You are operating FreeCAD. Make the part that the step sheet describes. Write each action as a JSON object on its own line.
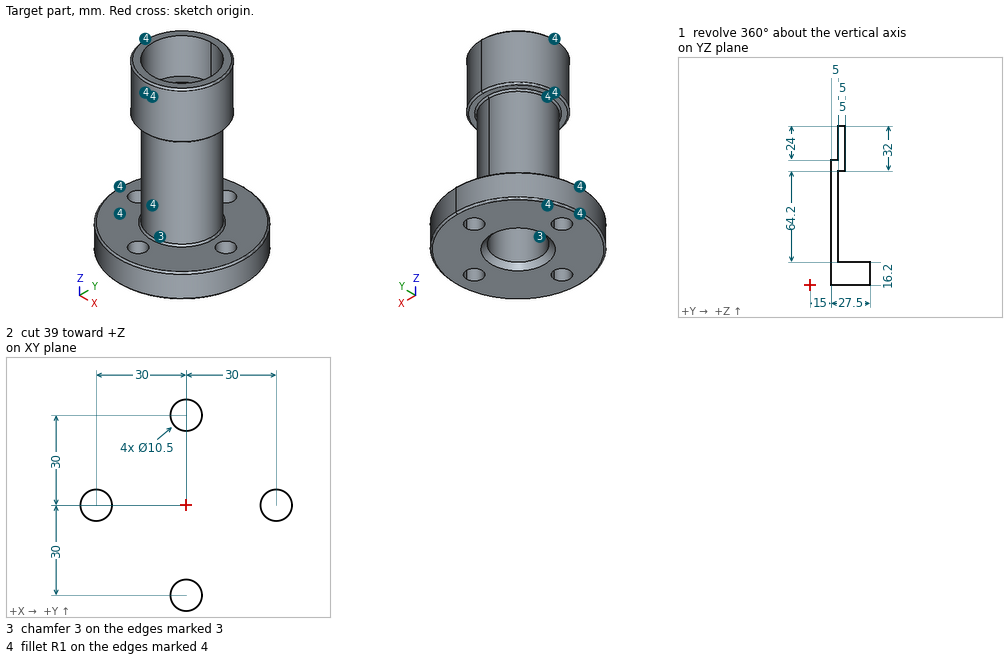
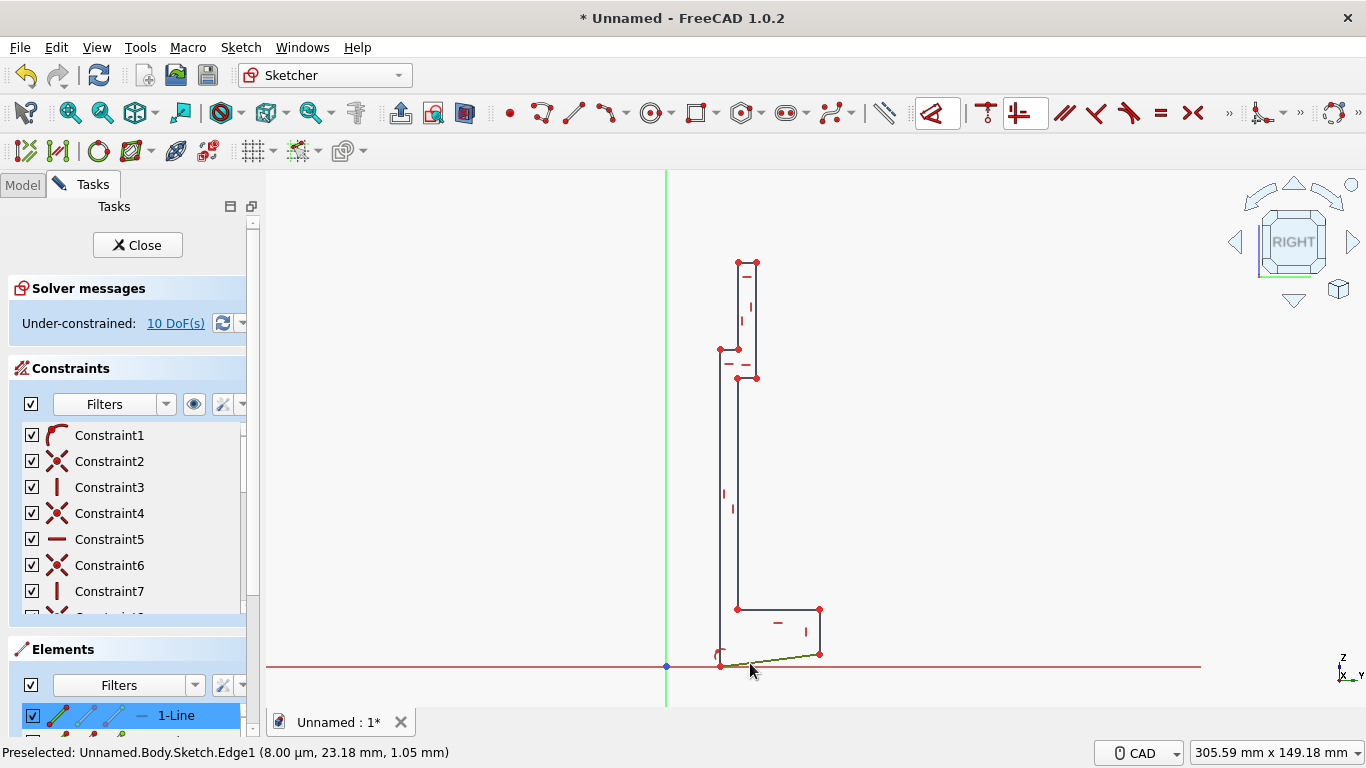
{"action": "left_click", "coordinate": [1042, 114]}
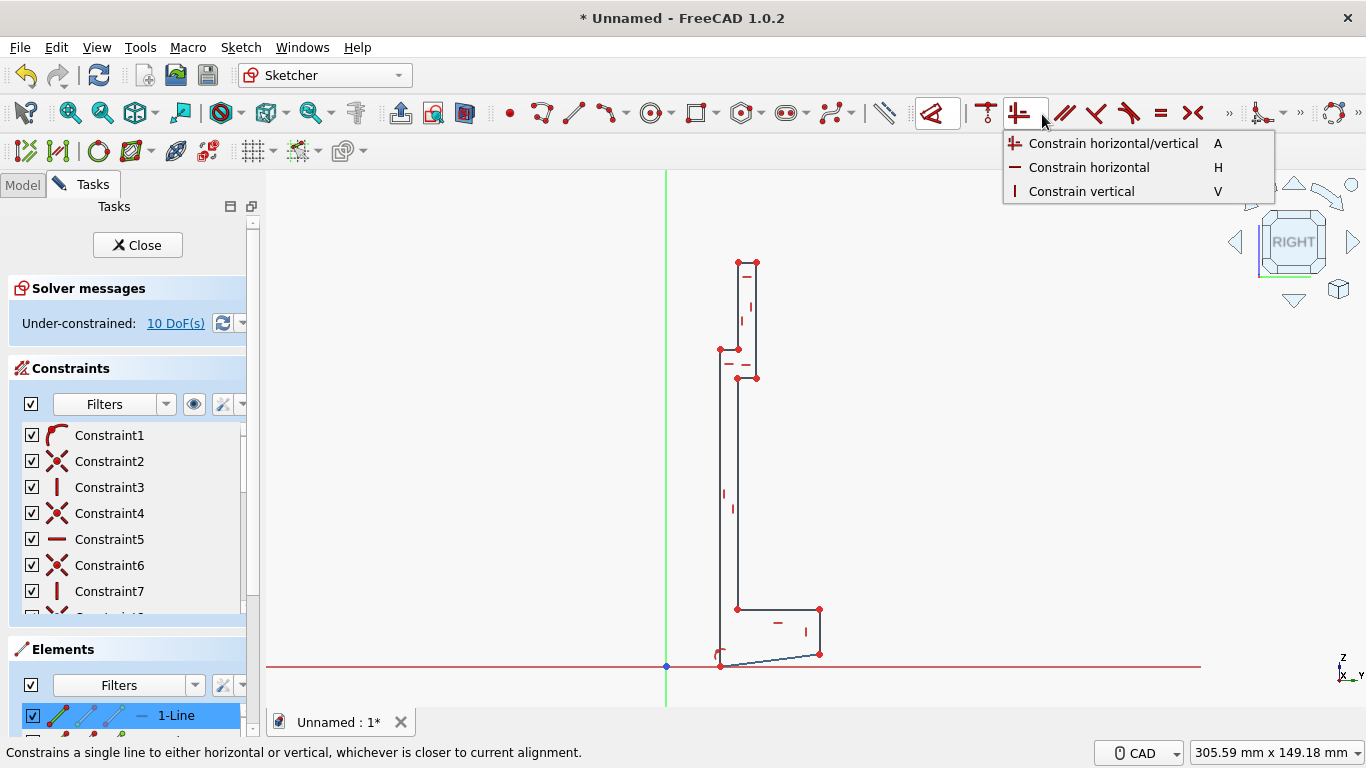
{"action": "left_click", "coordinate": [1139, 167]}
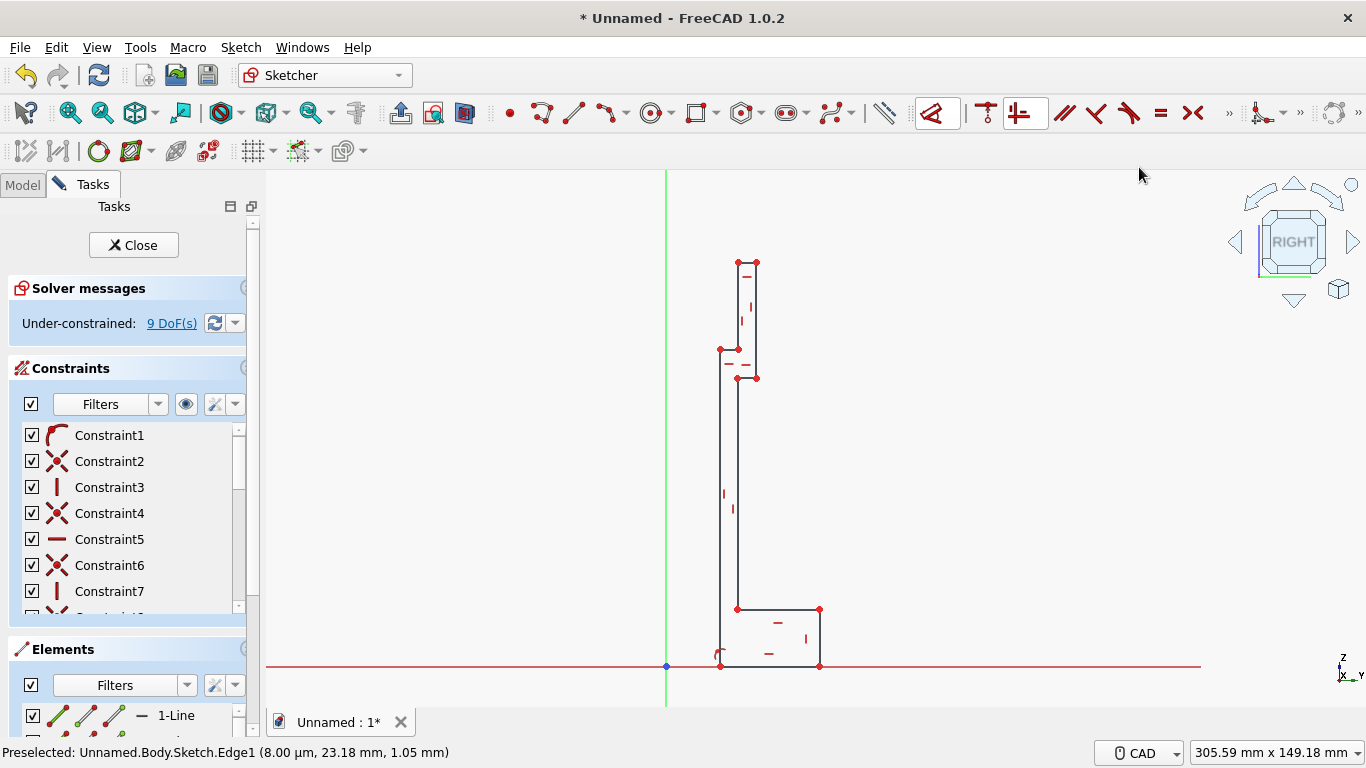
{"action": "left_click", "coordinate": [932, 114]}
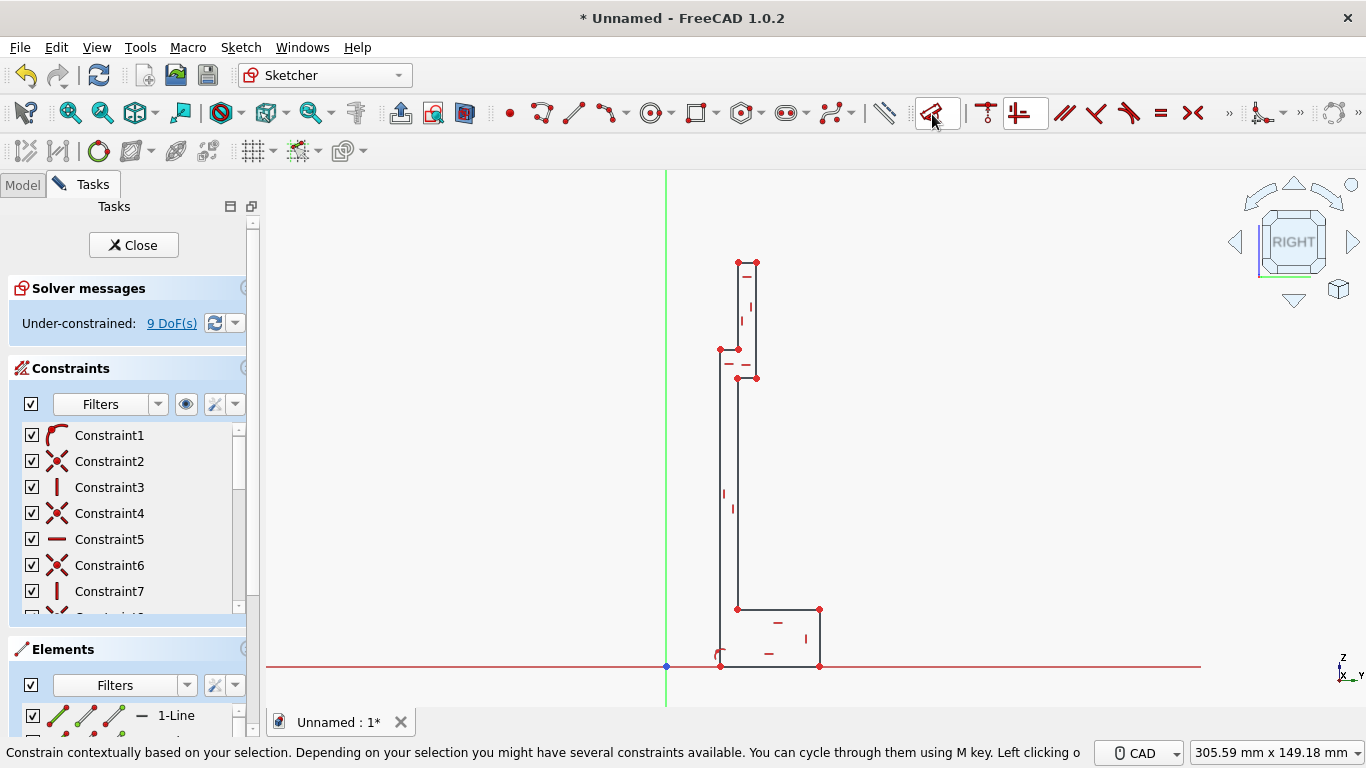
{"action": "scroll", "coordinate": [747, 378], "scroll_direction": "up", "scroll_amount": 4}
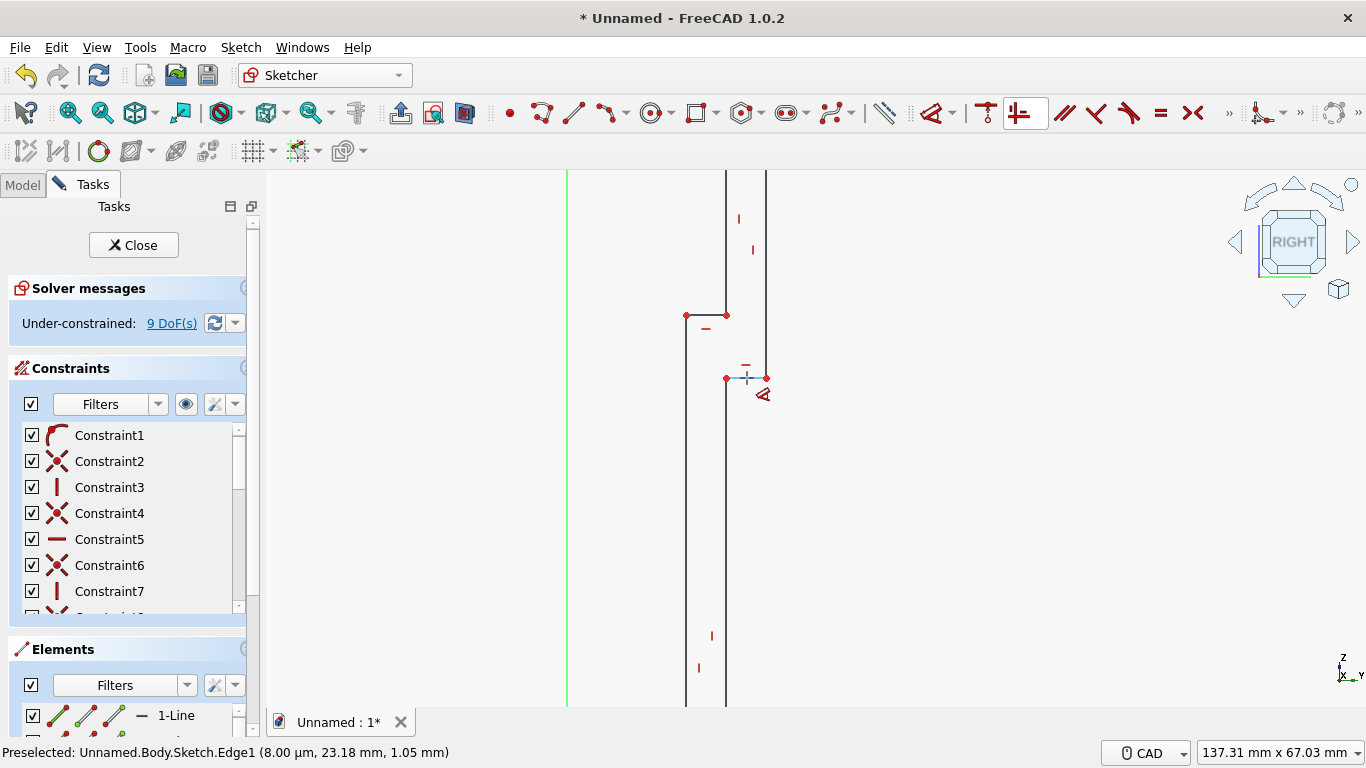
{"action": "left_click", "coordinate": [746, 378]}
{"action": "left_click", "coordinate": [746, 344]}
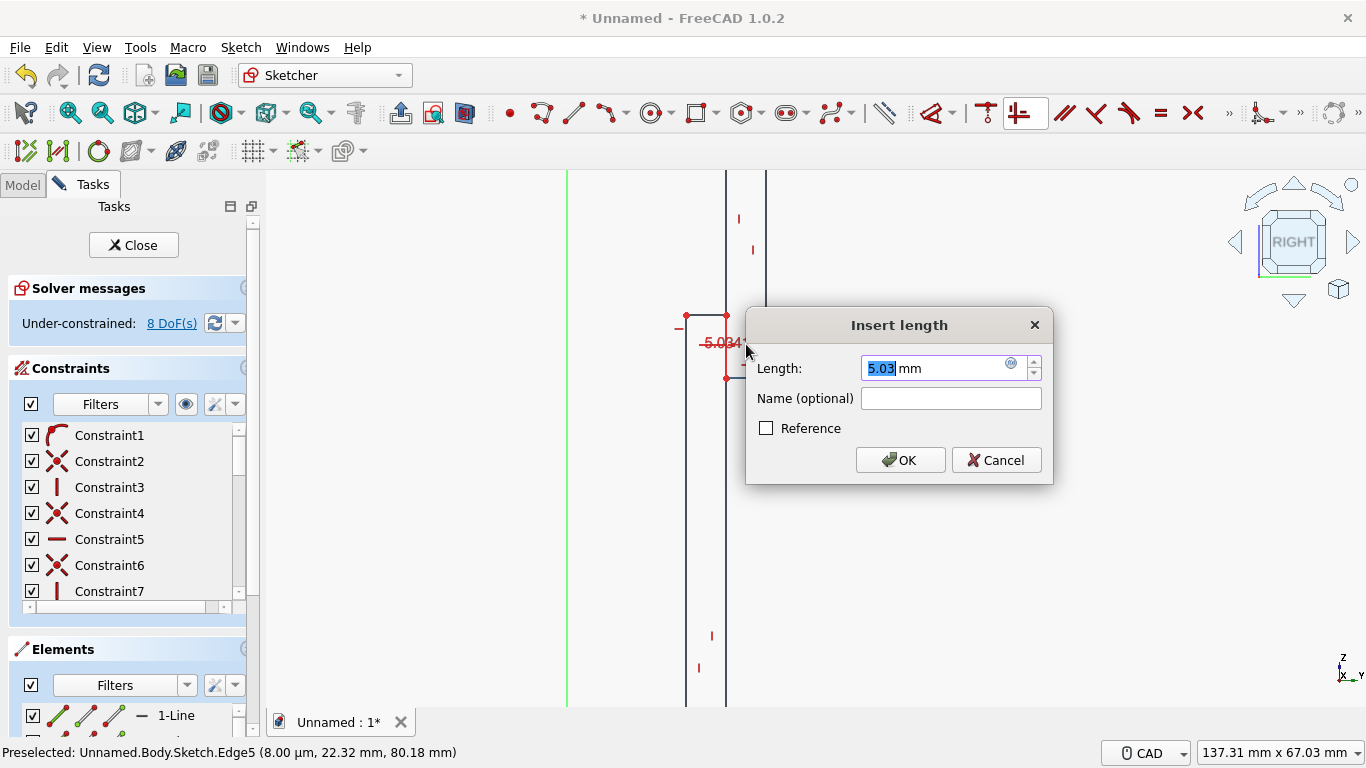
{"action": "type", "text": "5"}
{"action": "key", "text": "Return"}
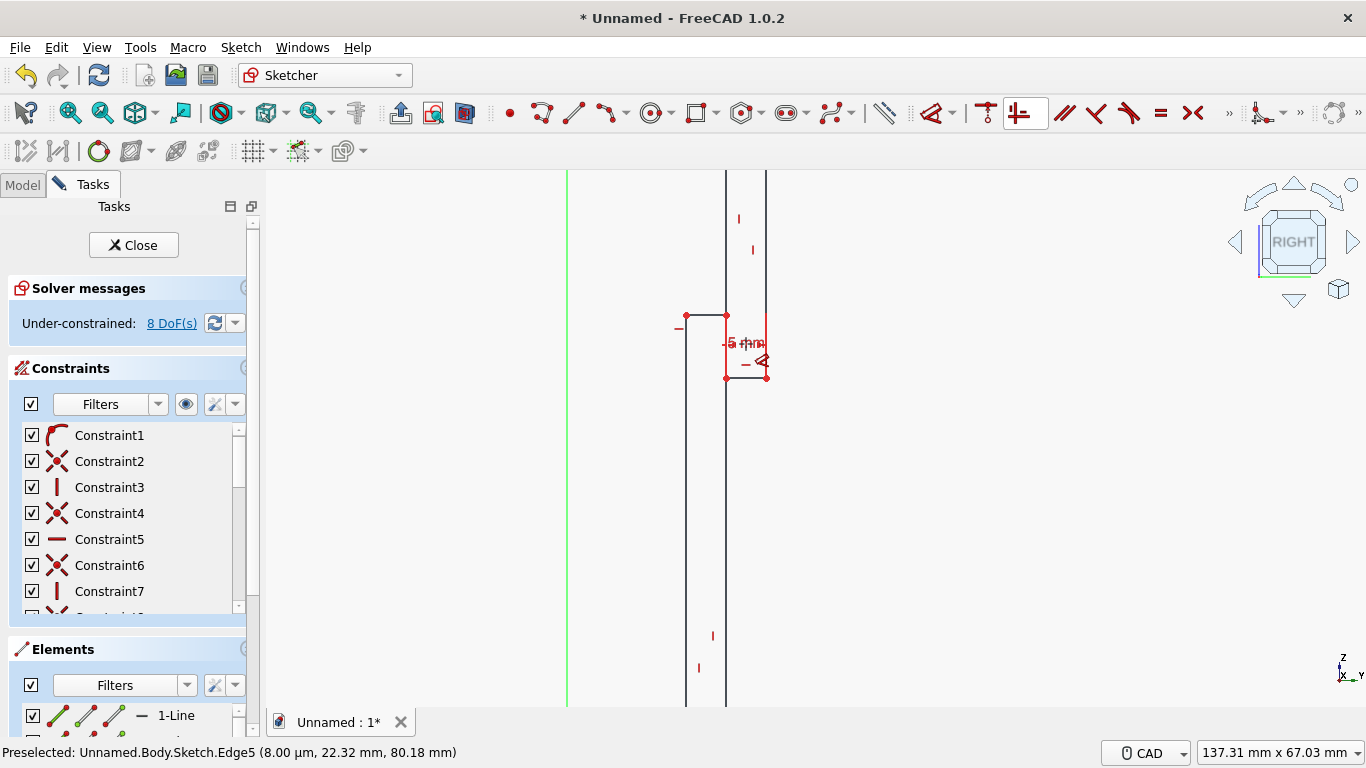
{"action": "scroll", "coordinate": [753, 362], "scroll_direction": "down", "scroll_amount": 5}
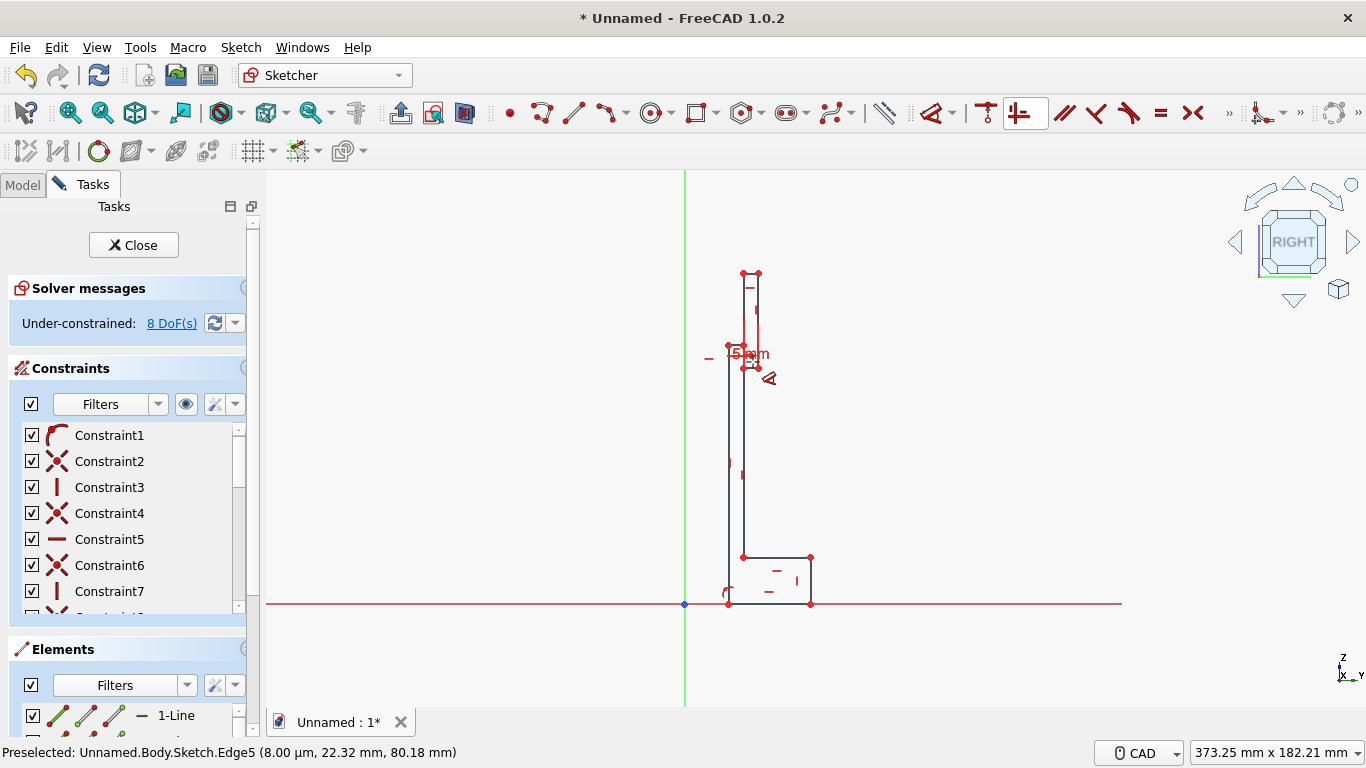
{"action": "scroll", "coordinate": [754, 274], "scroll_direction": "up", "scroll_amount": 6}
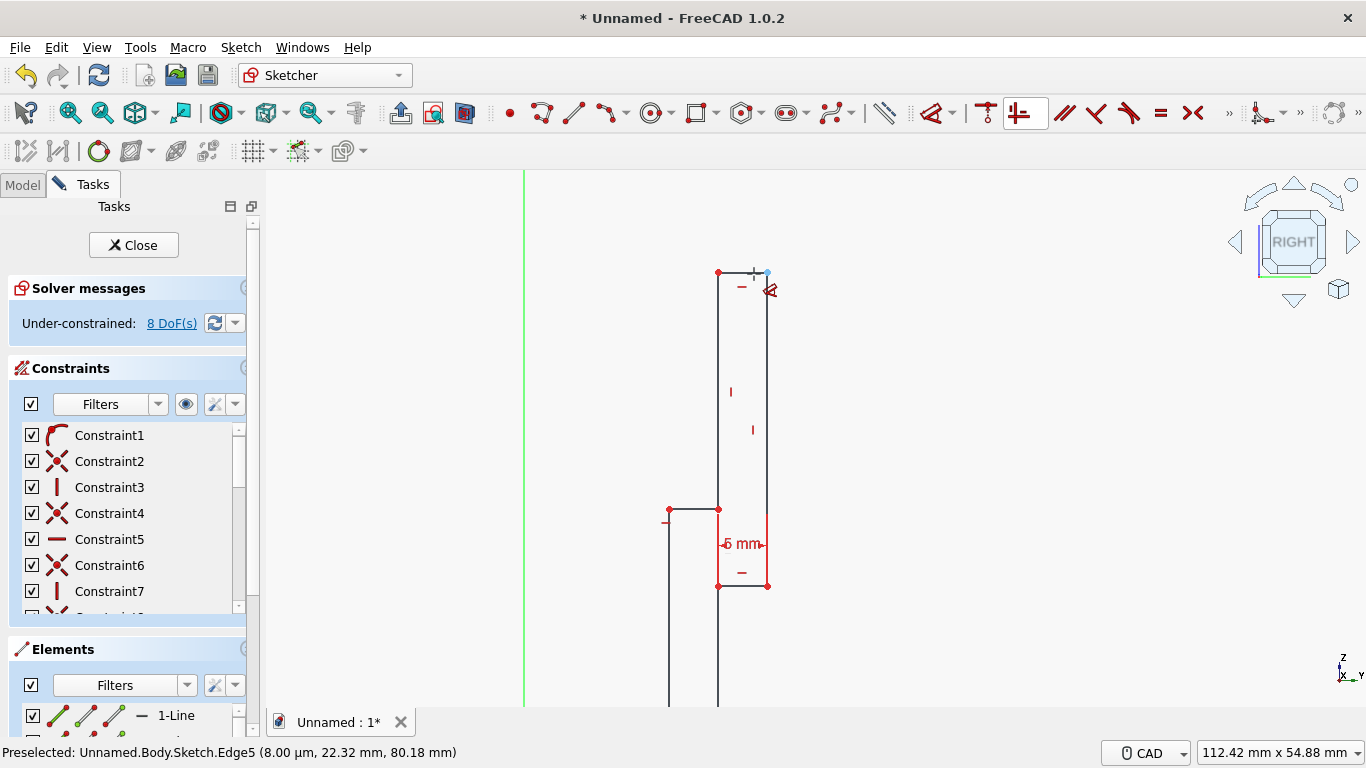
{"action": "left_click", "coordinate": [752, 273]}
{"action": "left_click", "coordinate": [743, 239]}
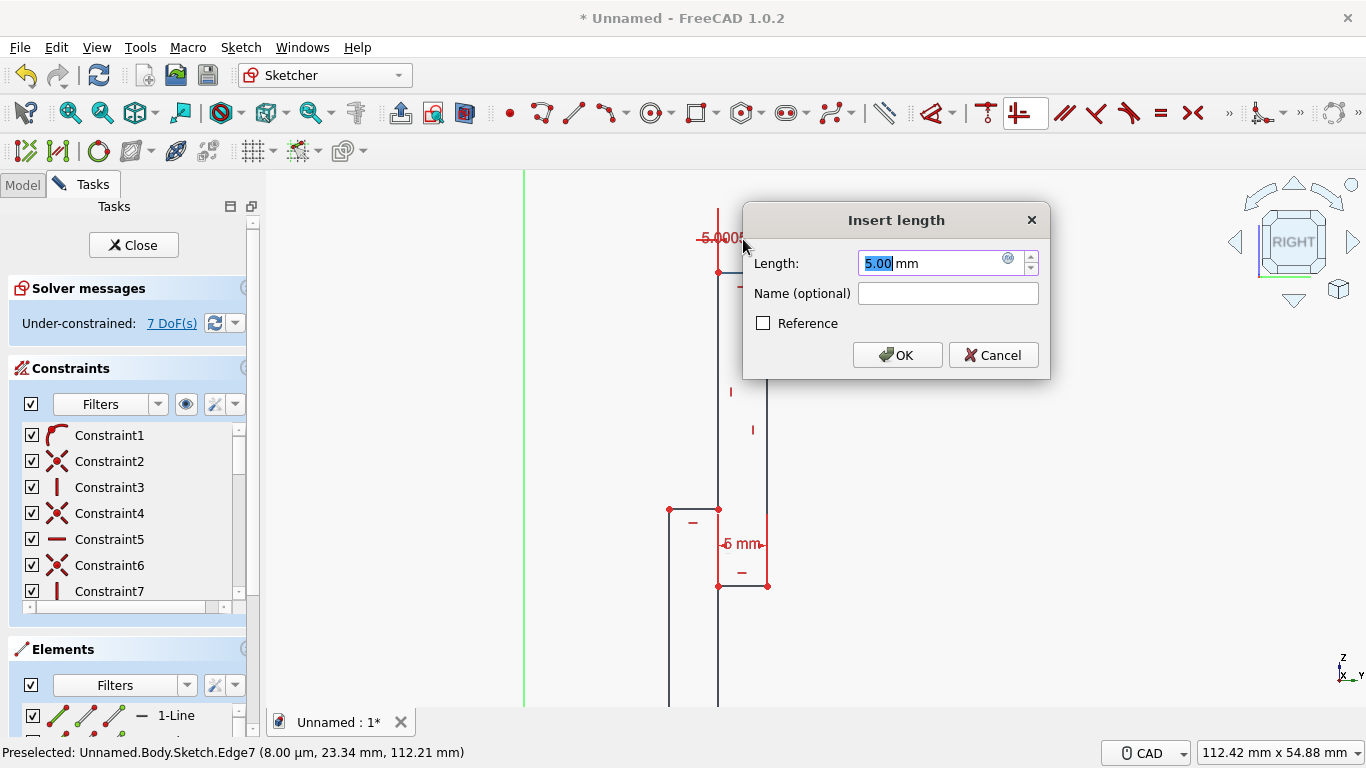
{"action": "type", "text": "5"}
{"action": "key", "text": "Return"}